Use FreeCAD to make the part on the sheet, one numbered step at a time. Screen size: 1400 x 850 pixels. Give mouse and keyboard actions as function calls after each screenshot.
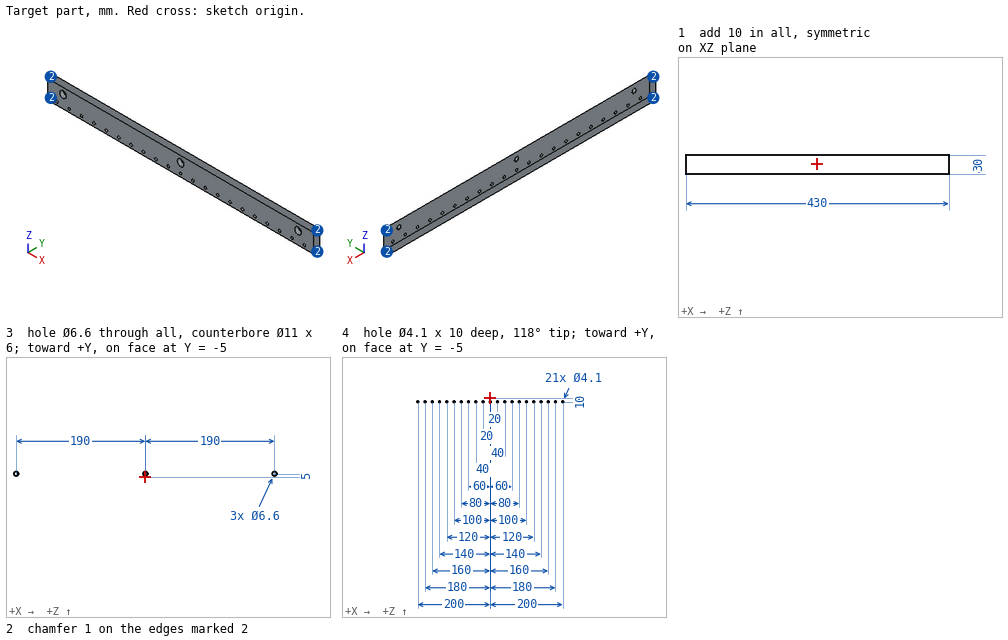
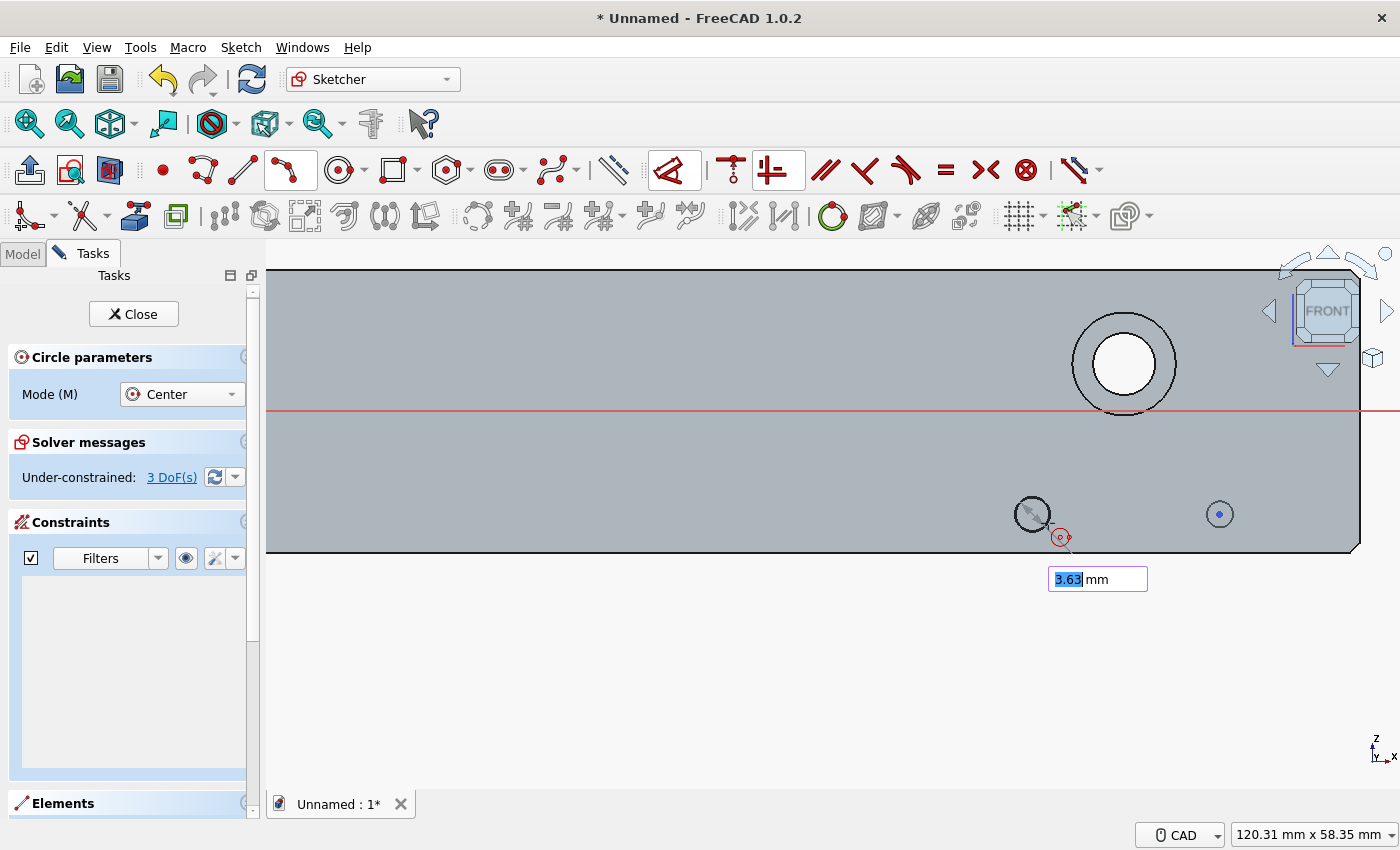
click(1044, 519)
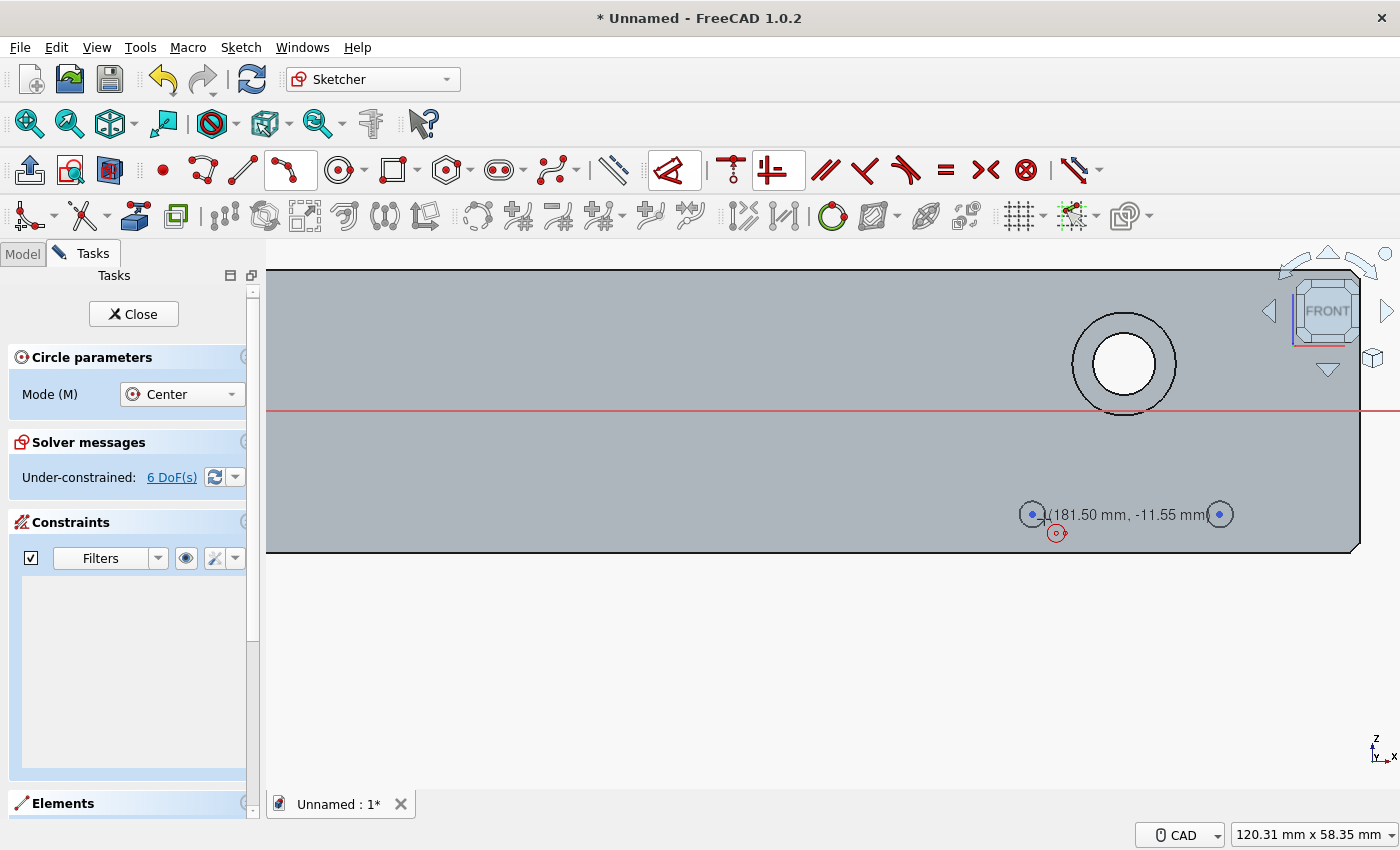
scroll(1048, 523, down, 9)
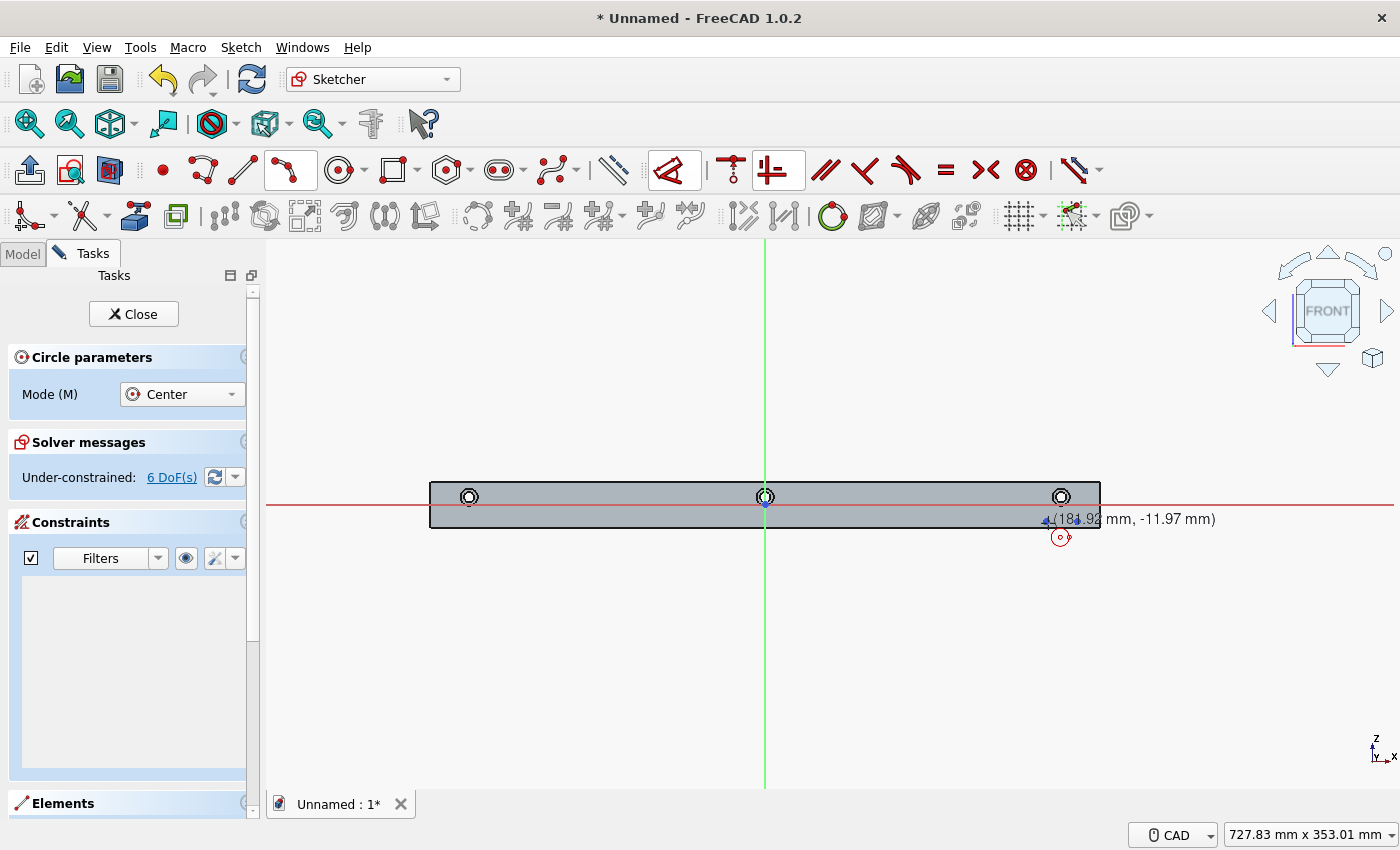
click(1014, 521)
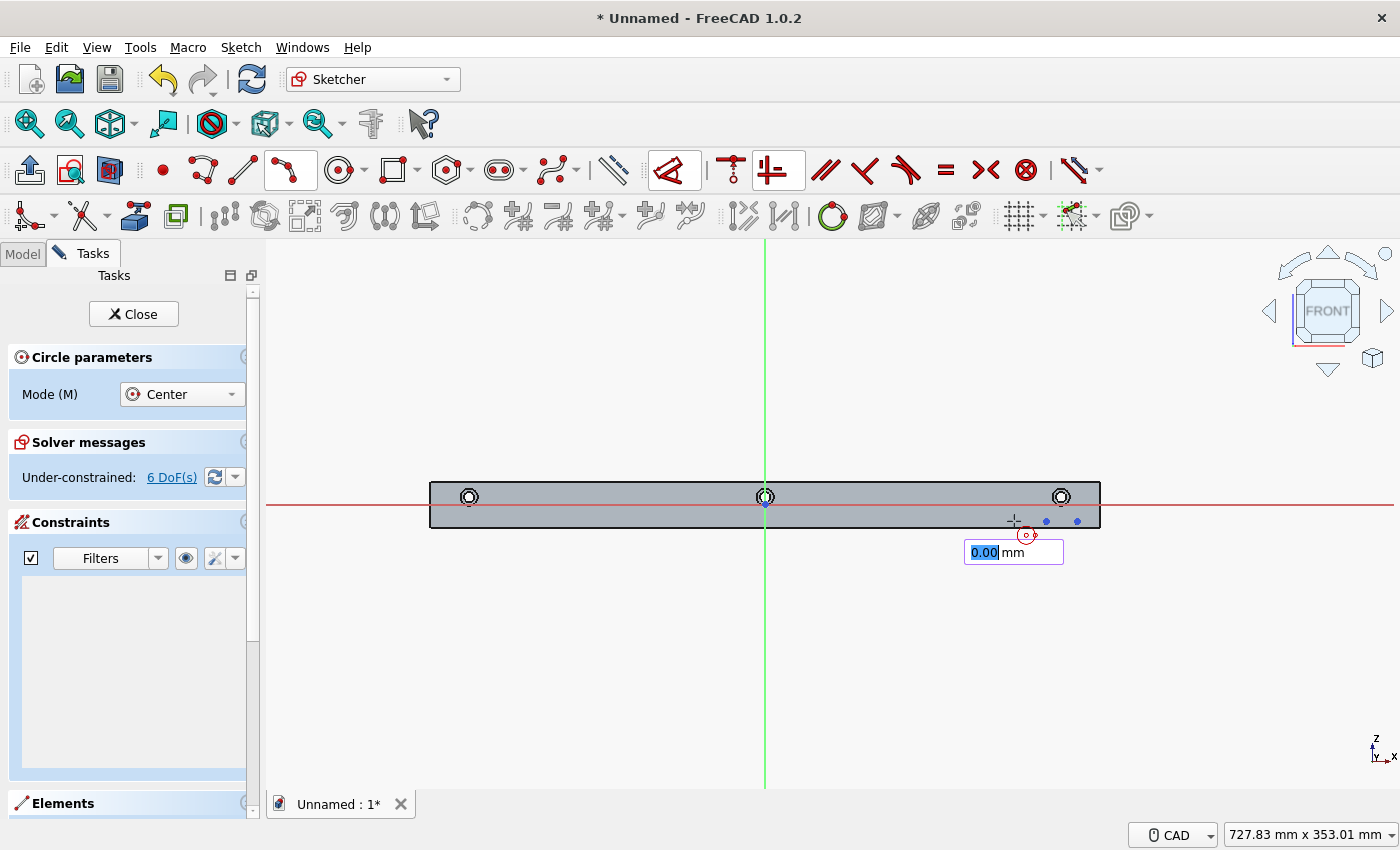
scroll(1017, 523, up, 9)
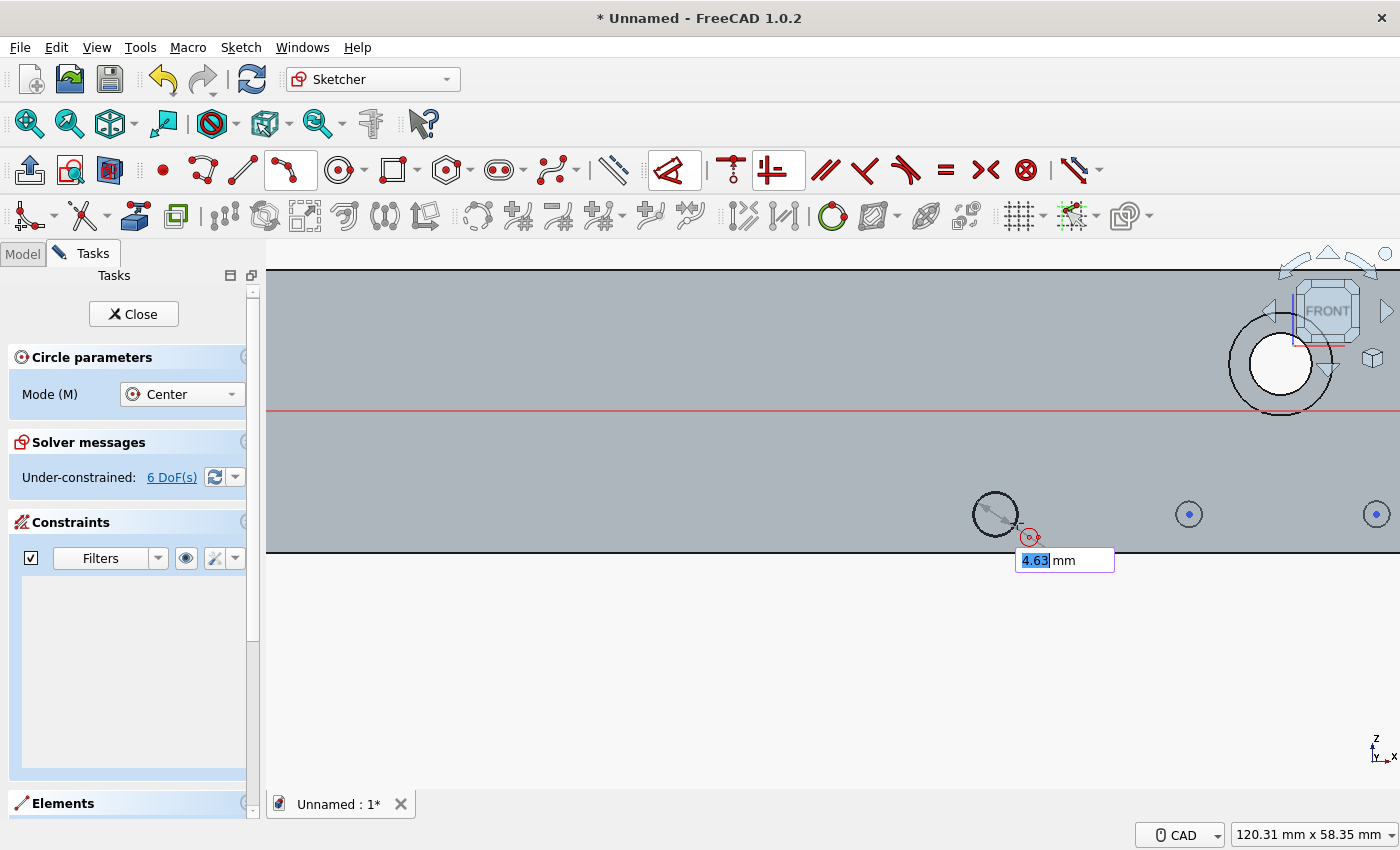
click(1012, 519)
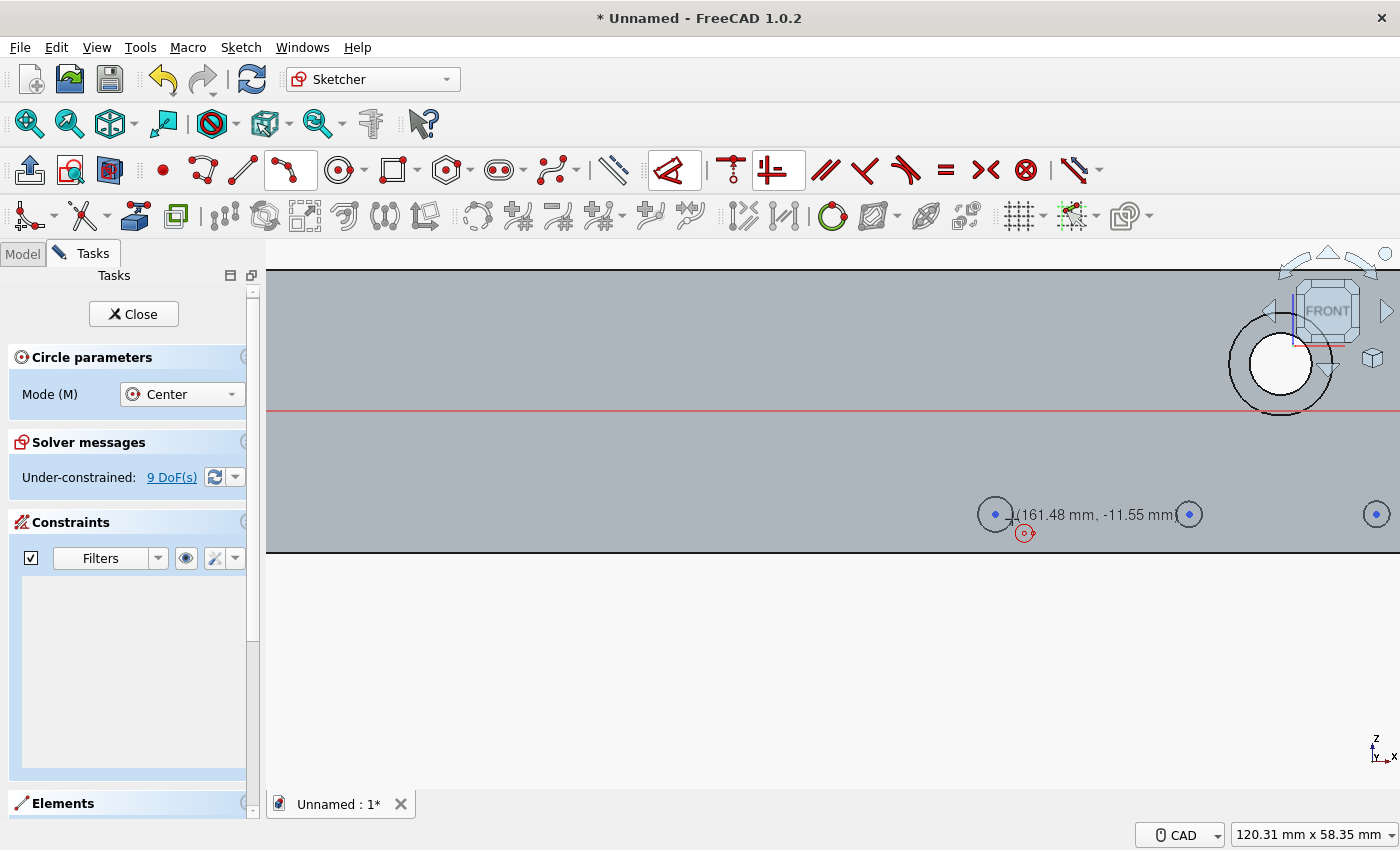
scroll(1017, 523, down, 9)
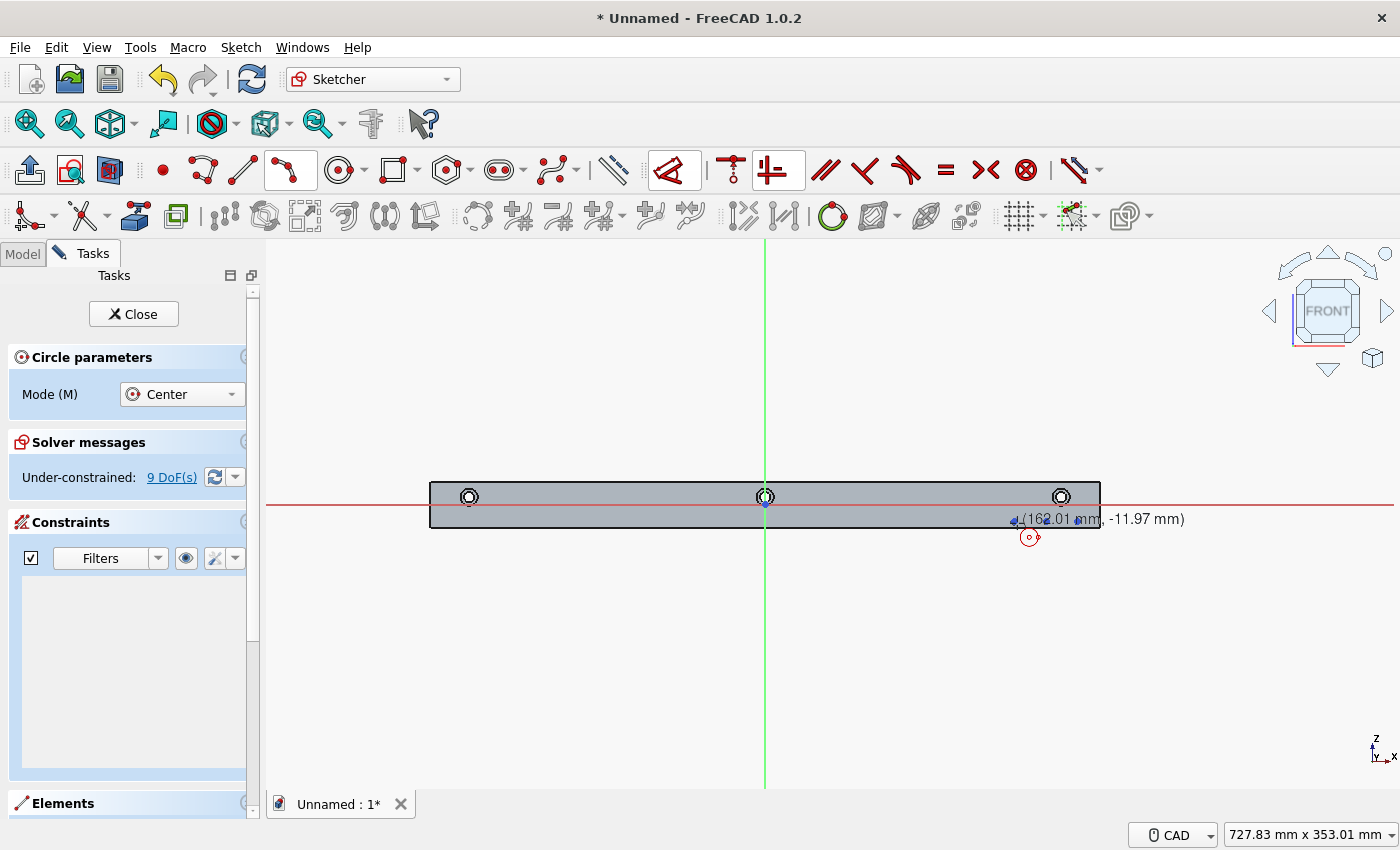
click(983, 521)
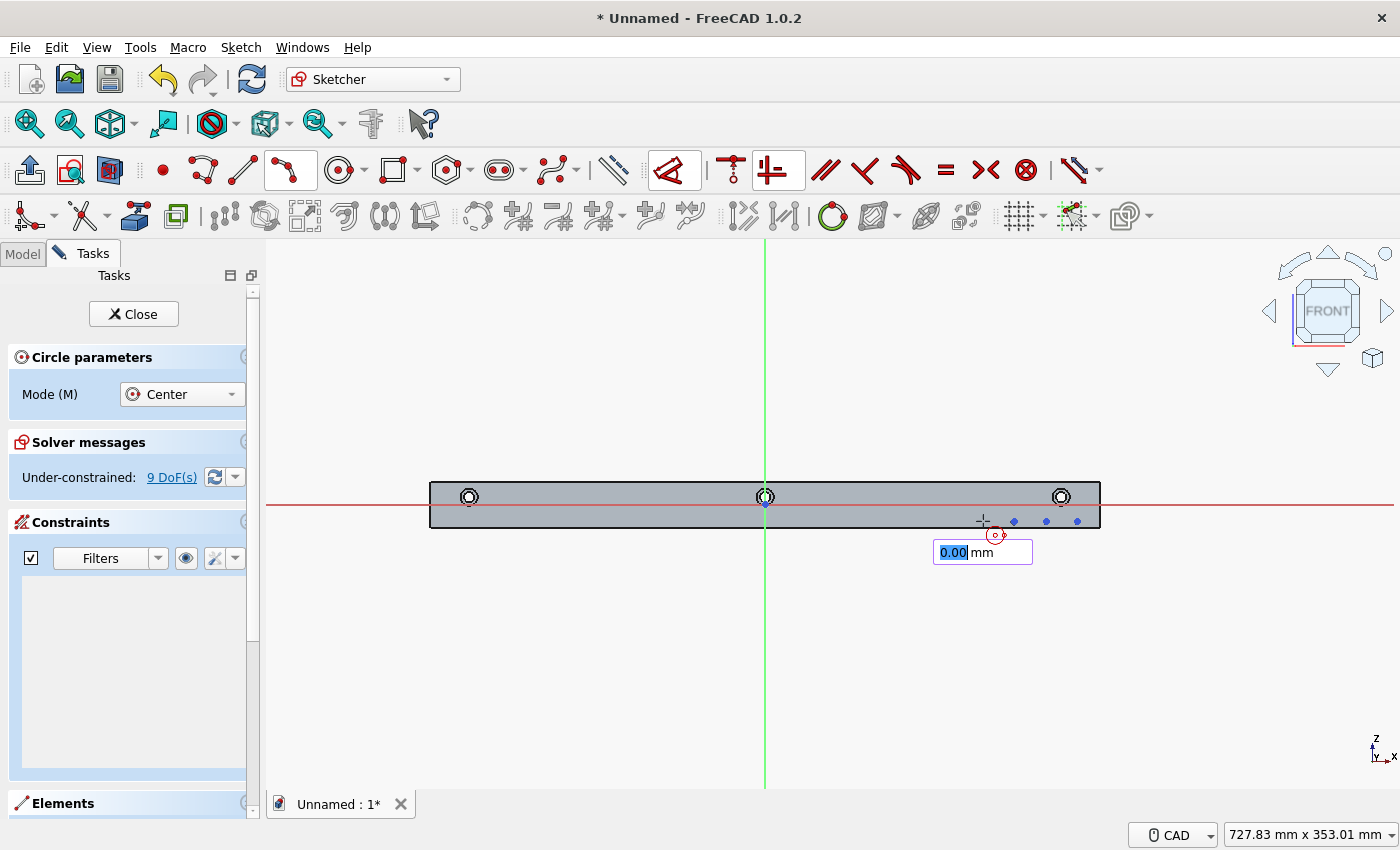
scroll(986, 523, up, 9)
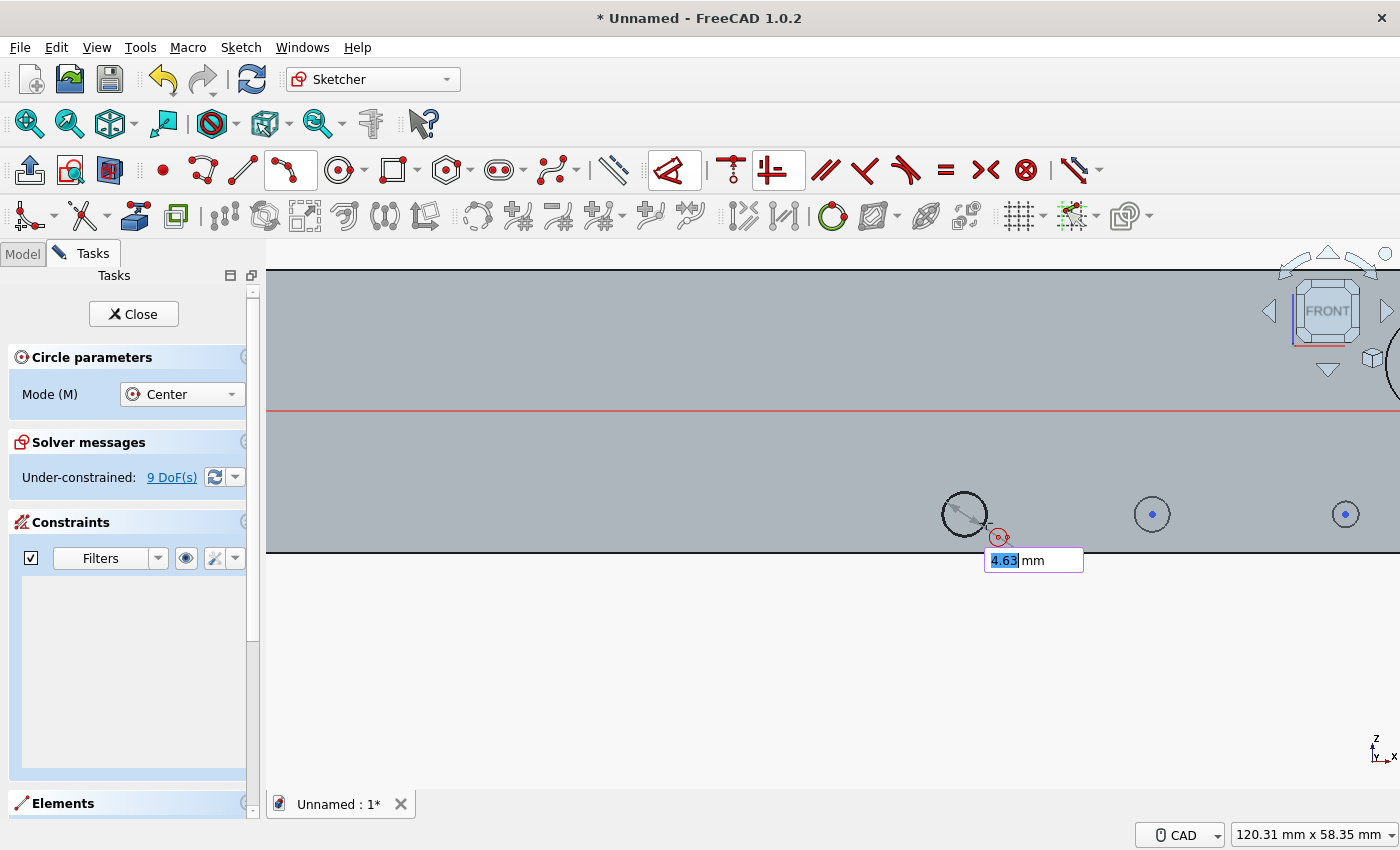
click(980, 519)